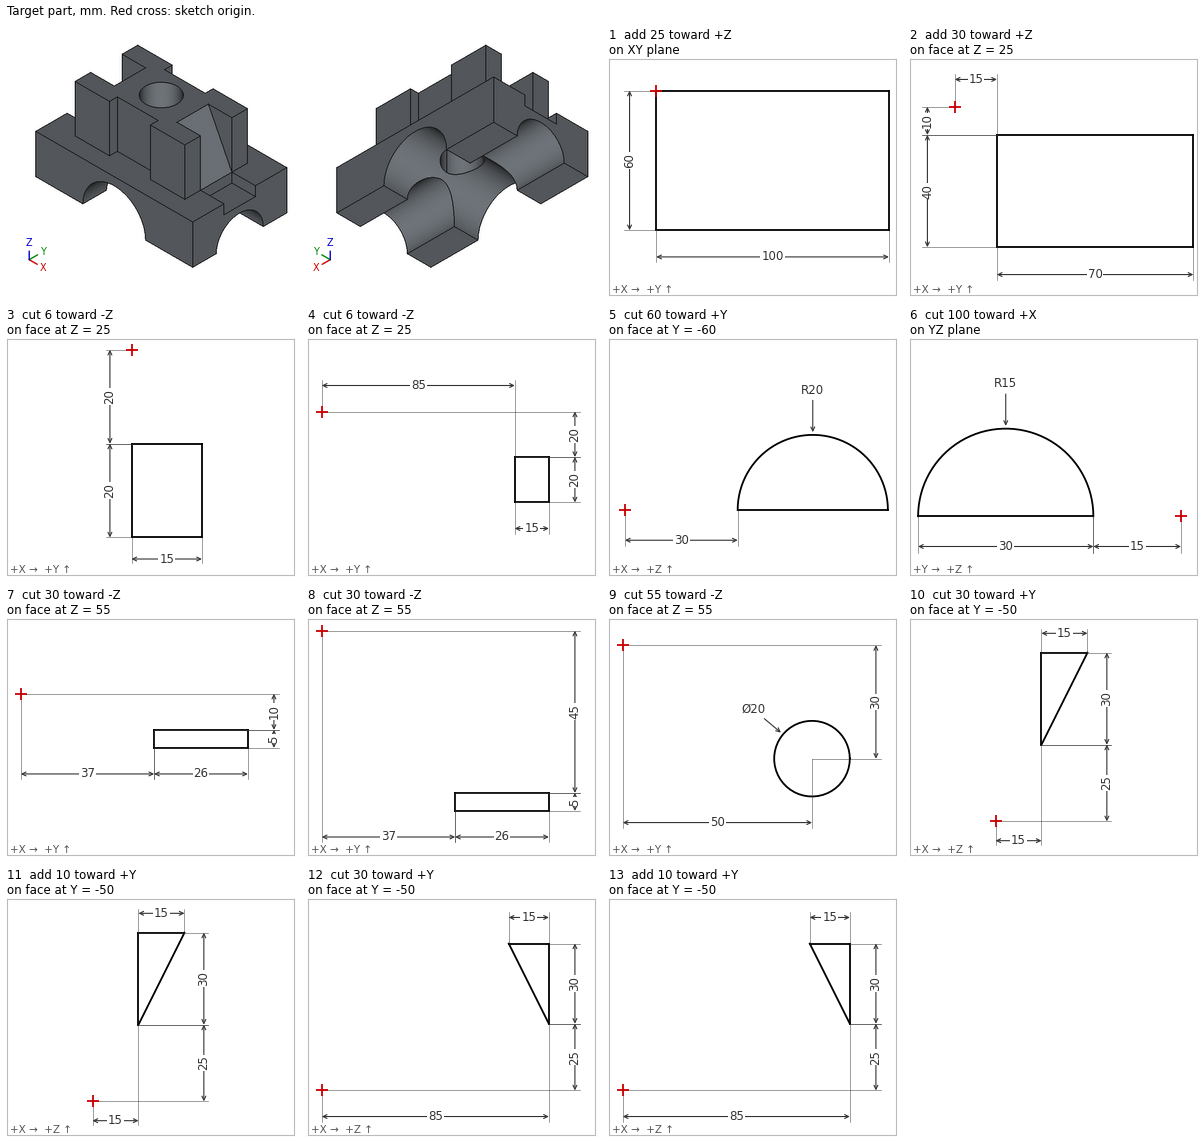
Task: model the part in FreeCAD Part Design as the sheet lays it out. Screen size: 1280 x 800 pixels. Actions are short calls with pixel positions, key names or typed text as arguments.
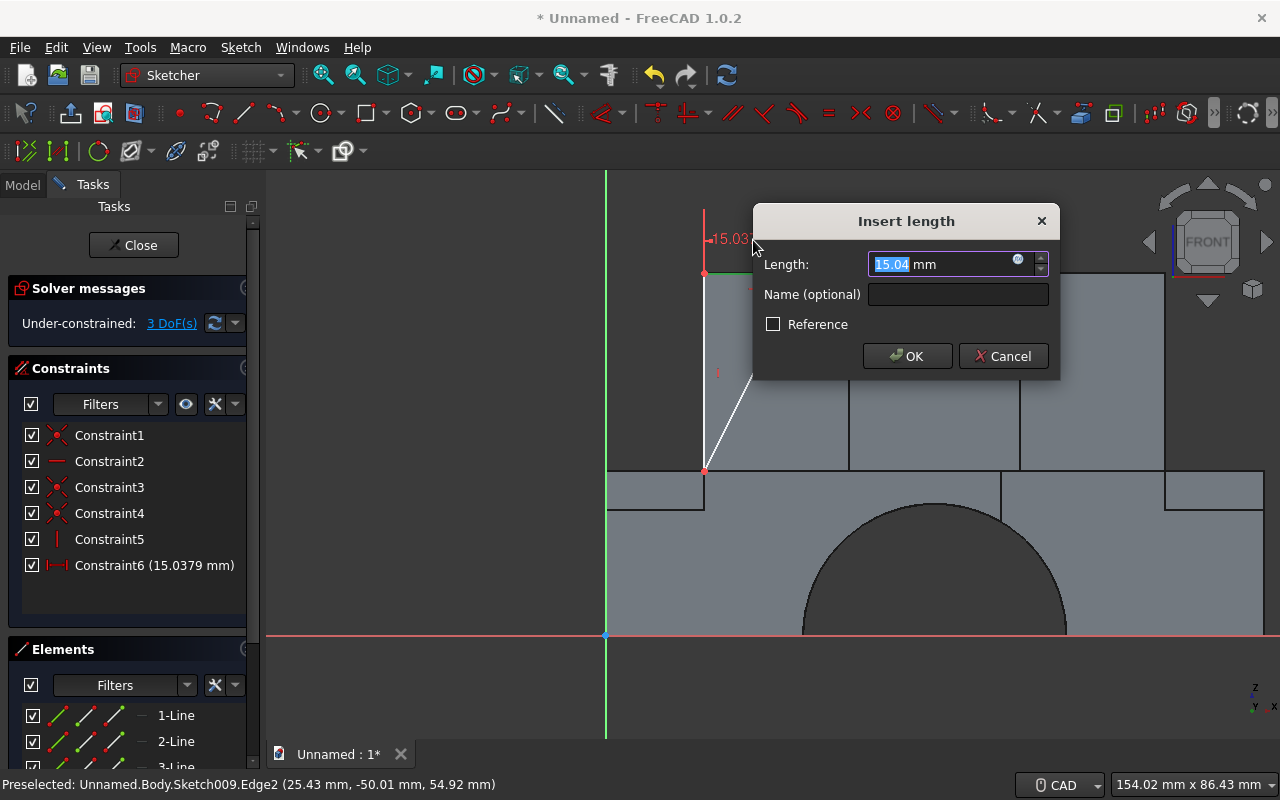
text(15)
key(Return)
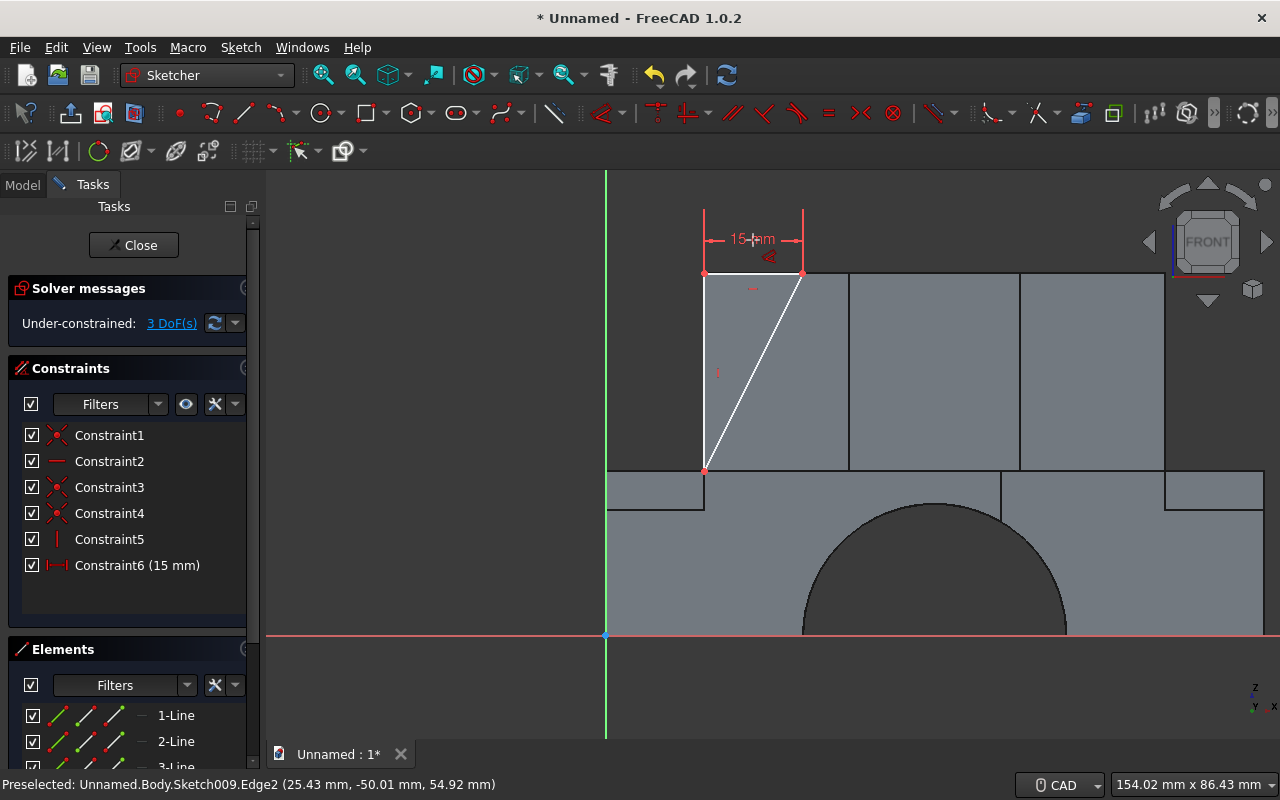
click(704, 333)
click(670, 373)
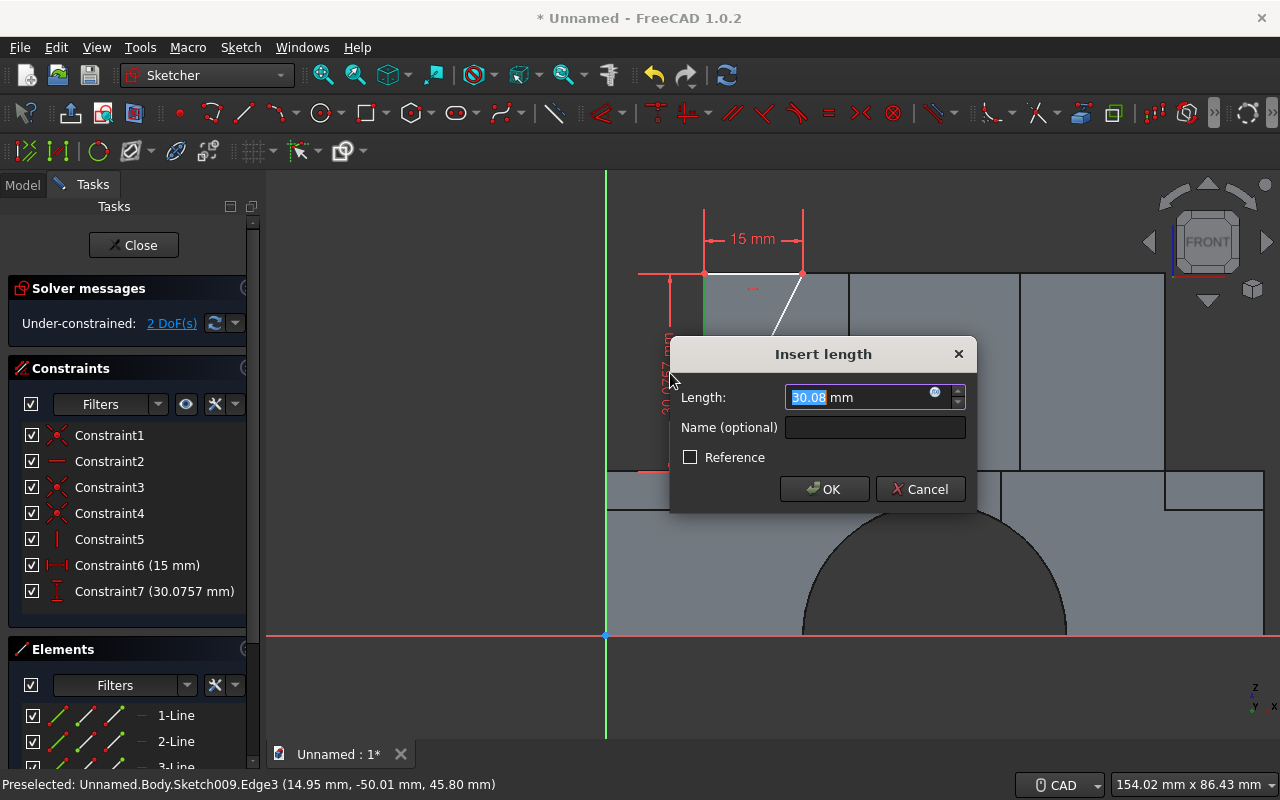
text(30)
key(Return)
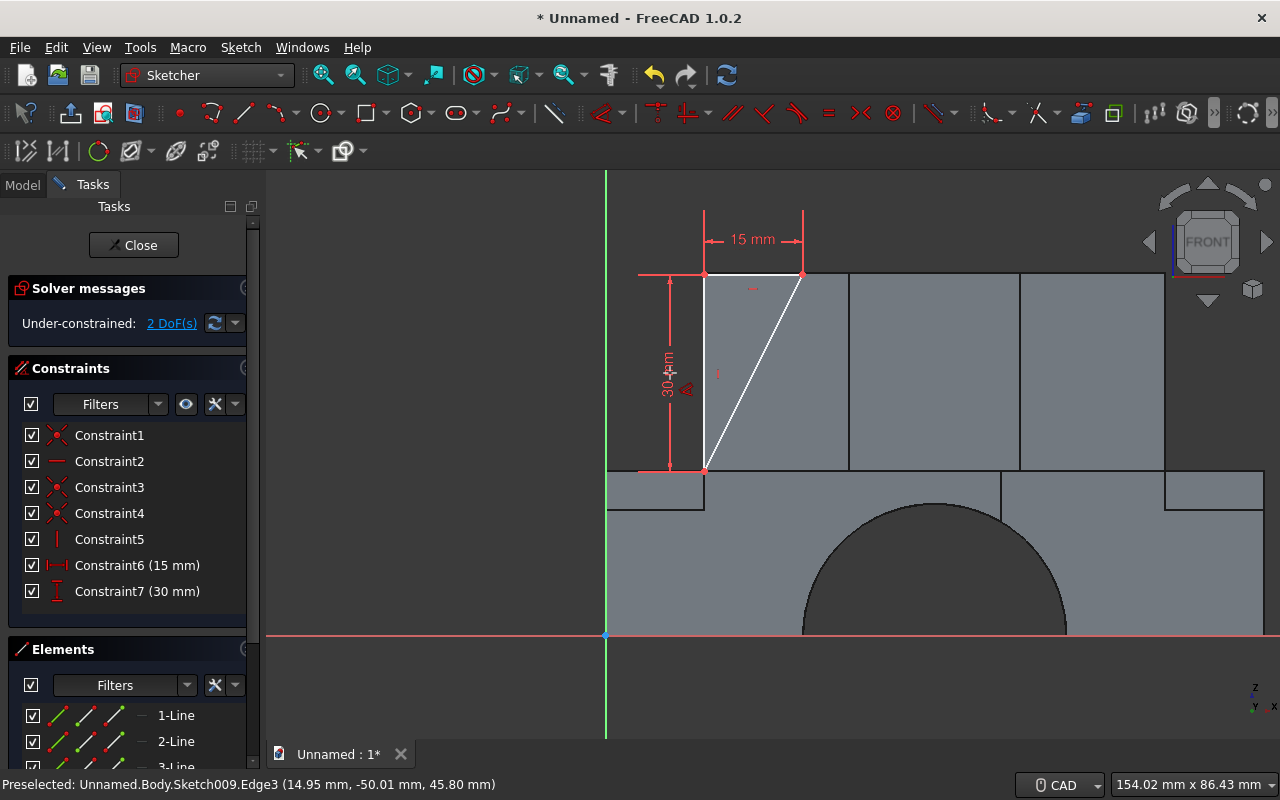
click(704, 472)
click(655, 670)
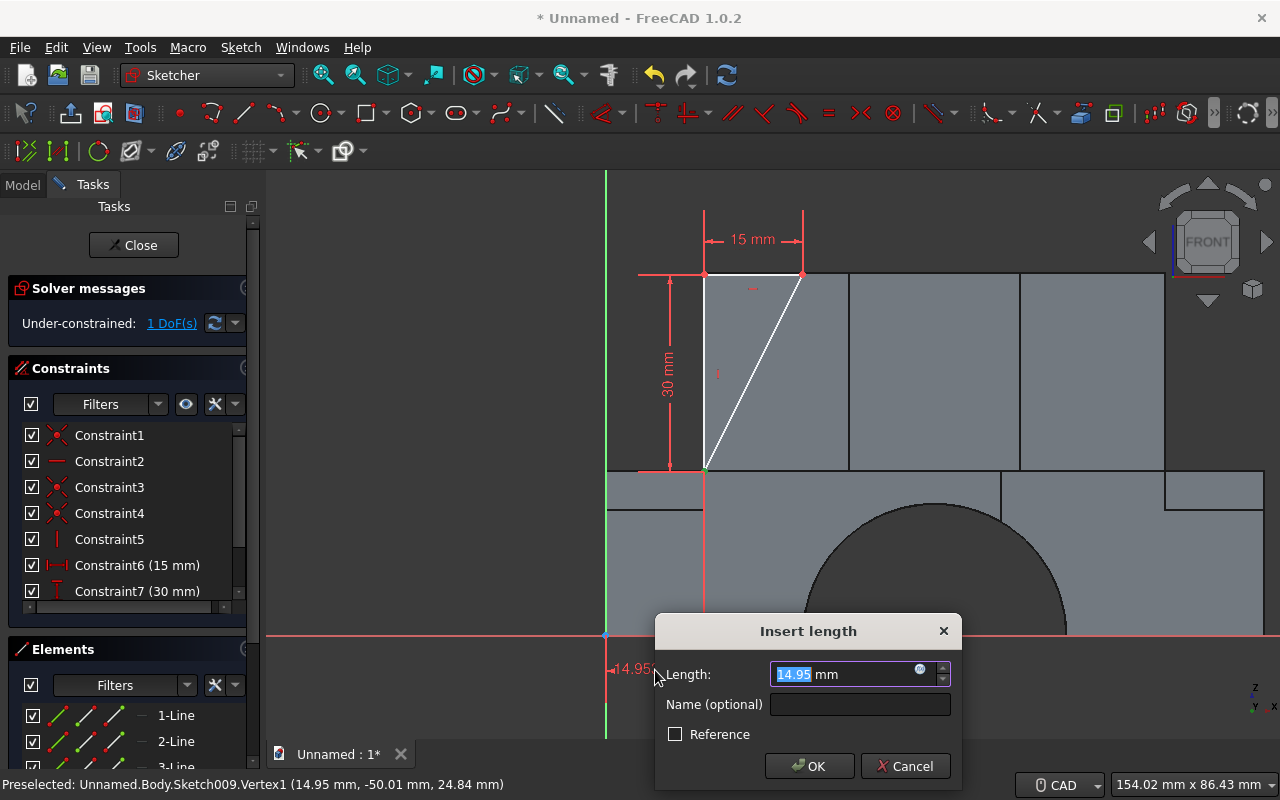
text(15)
key(Return)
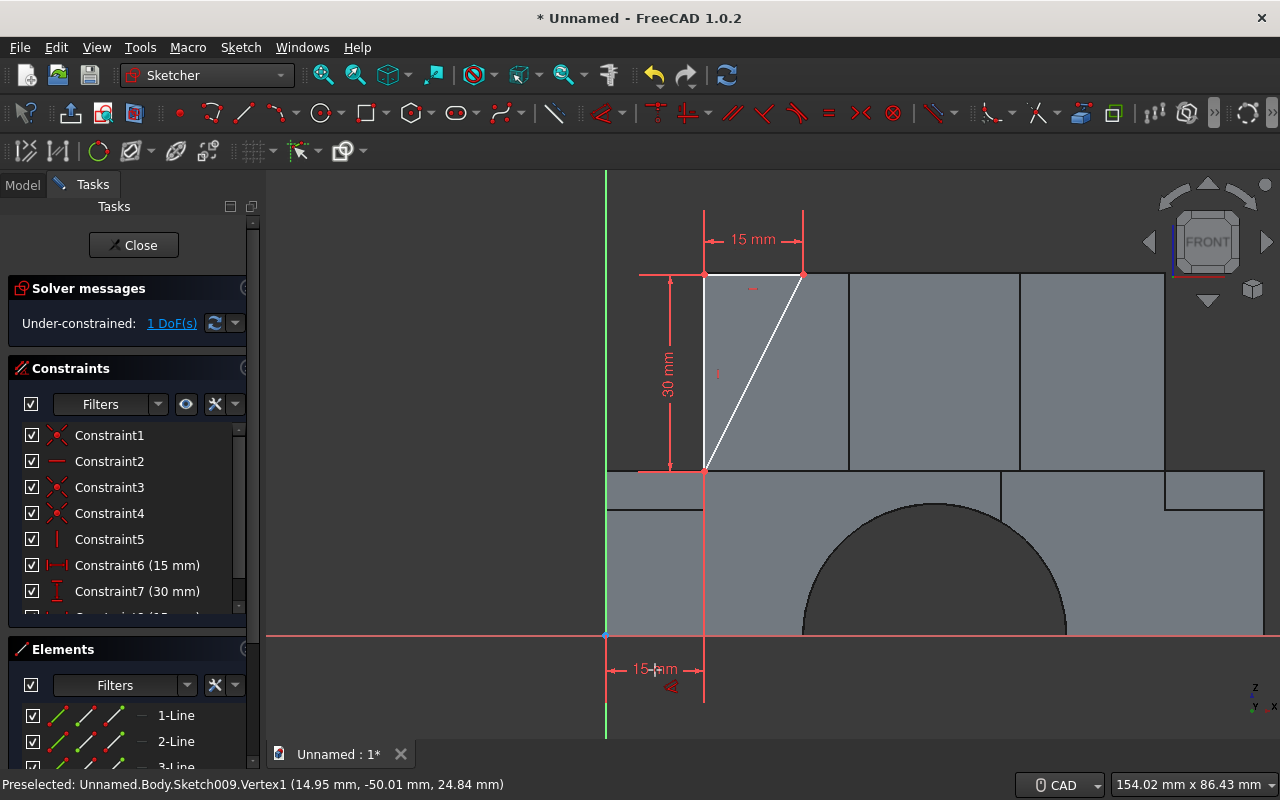
click(704, 472)
click(572, 554)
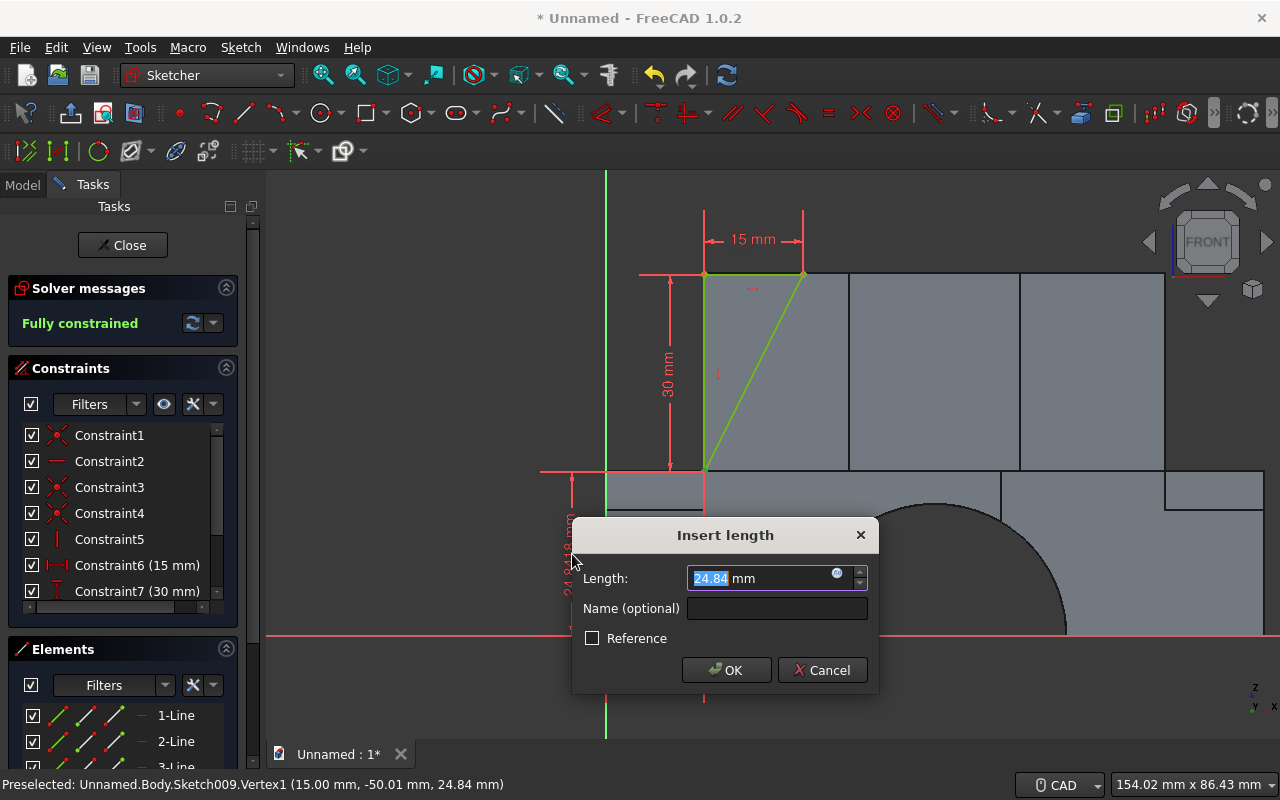
text(25)
key(Return)
key(Escape)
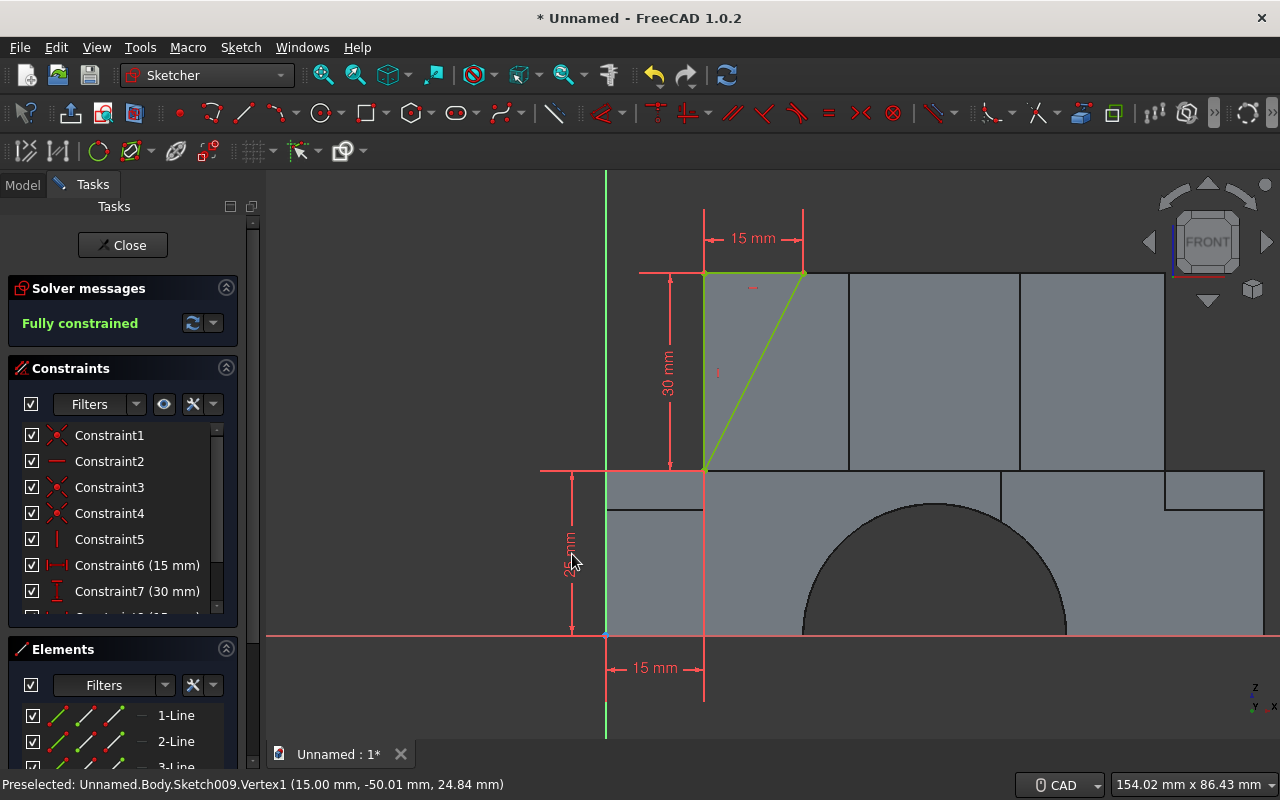
click(123, 245)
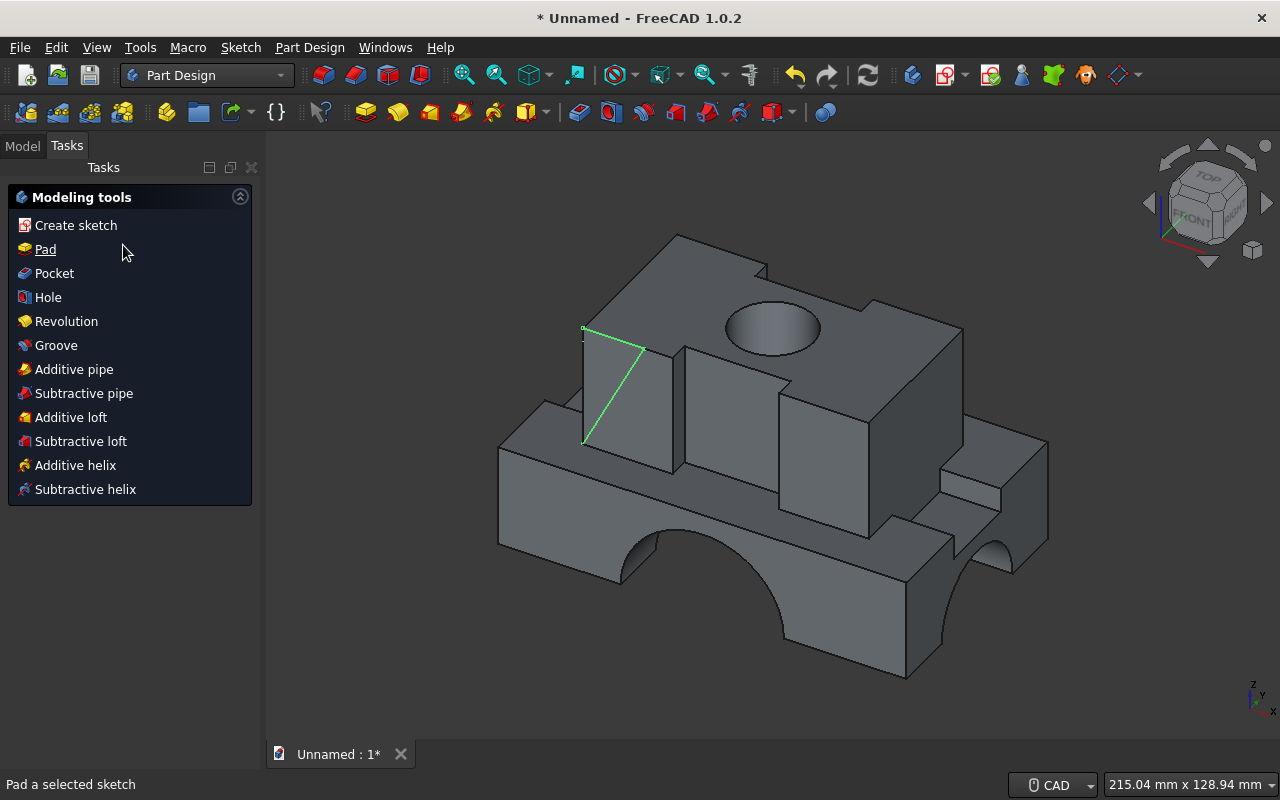
click(580, 112)